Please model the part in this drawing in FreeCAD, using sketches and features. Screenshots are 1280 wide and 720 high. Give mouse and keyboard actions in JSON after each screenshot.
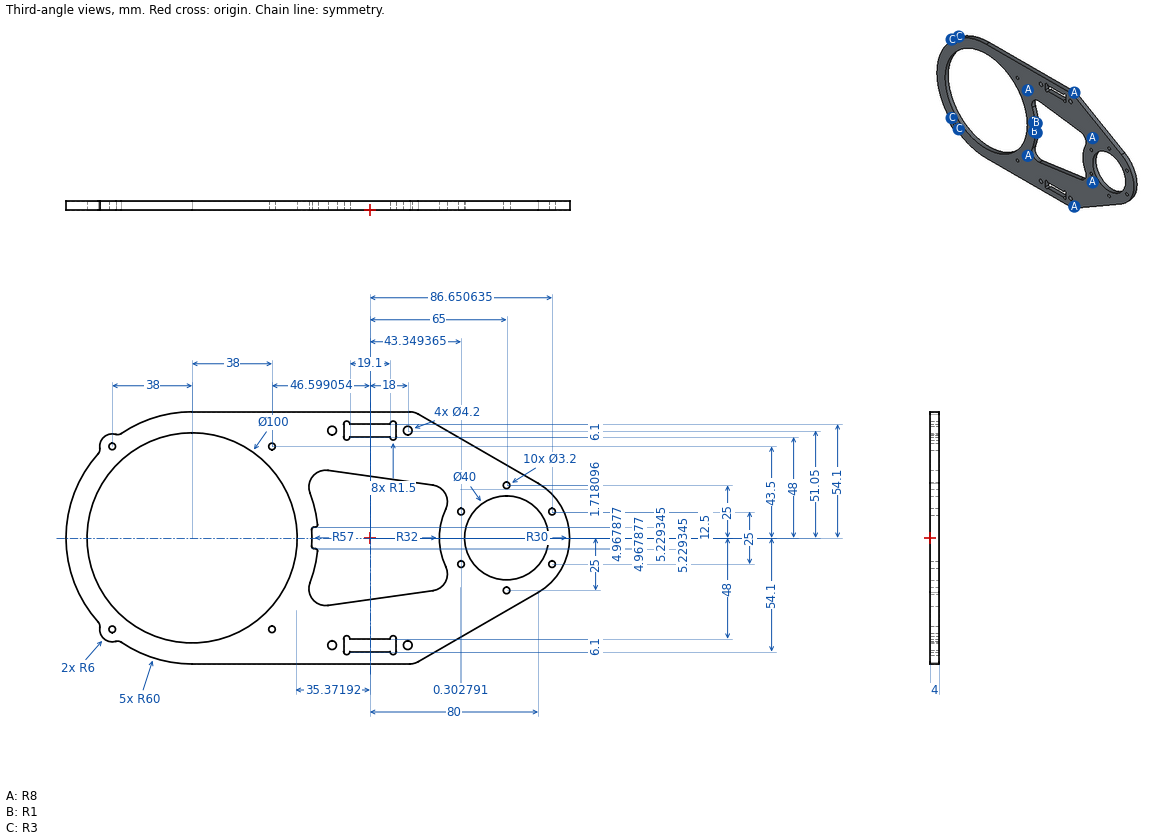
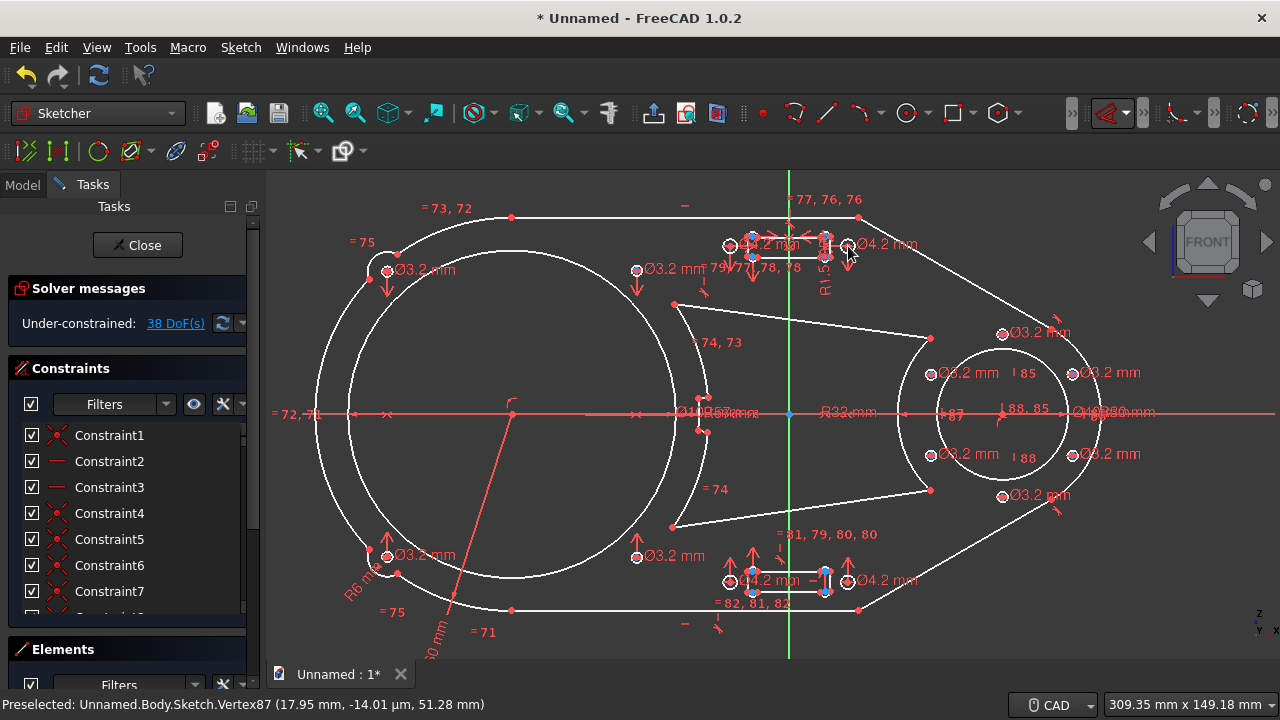
{"action": "left_click", "coordinate": [1128, 114]}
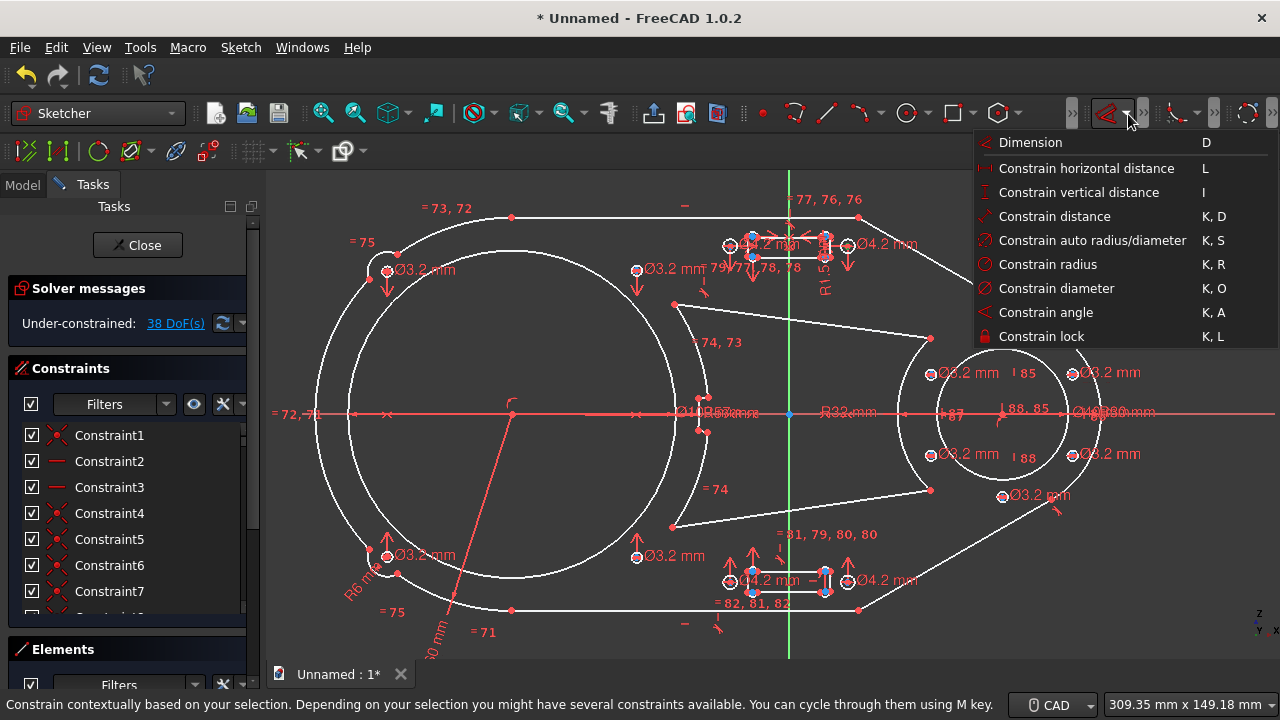
{"action": "left_click", "coordinate": [1126, 168]}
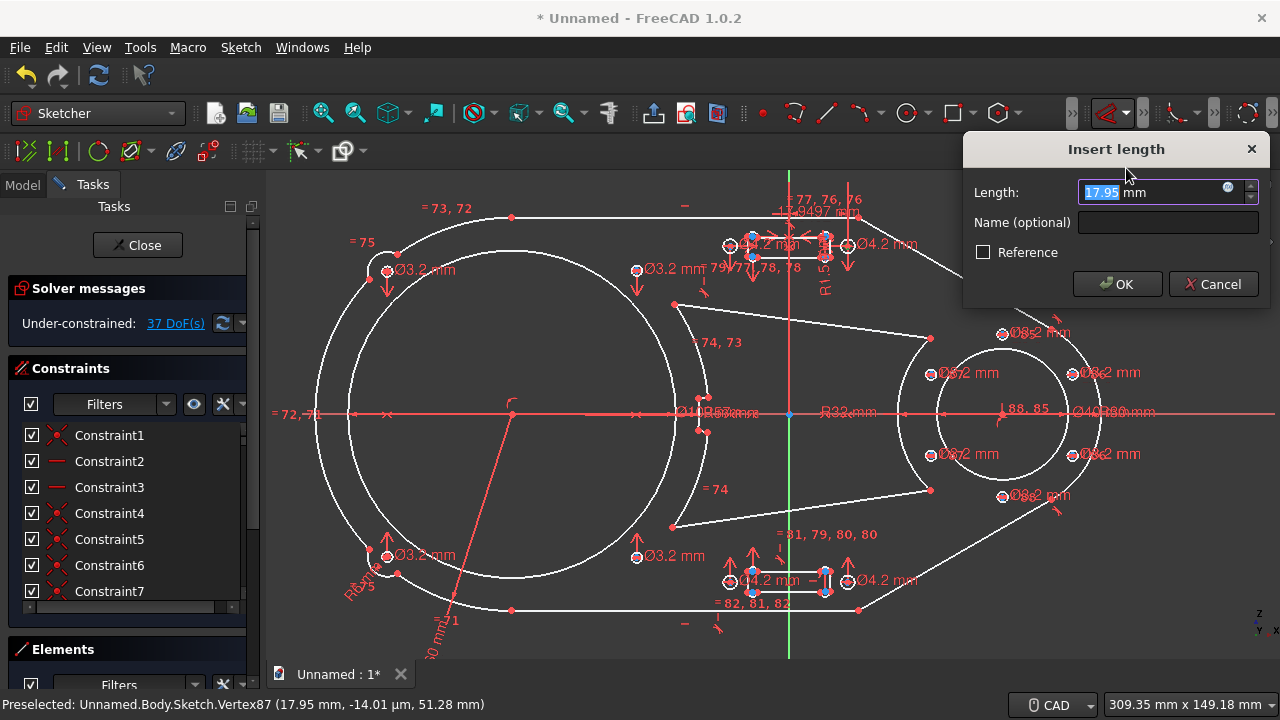
{"action": "type", "text": "18"}
{"action": "key", "text": "Return"}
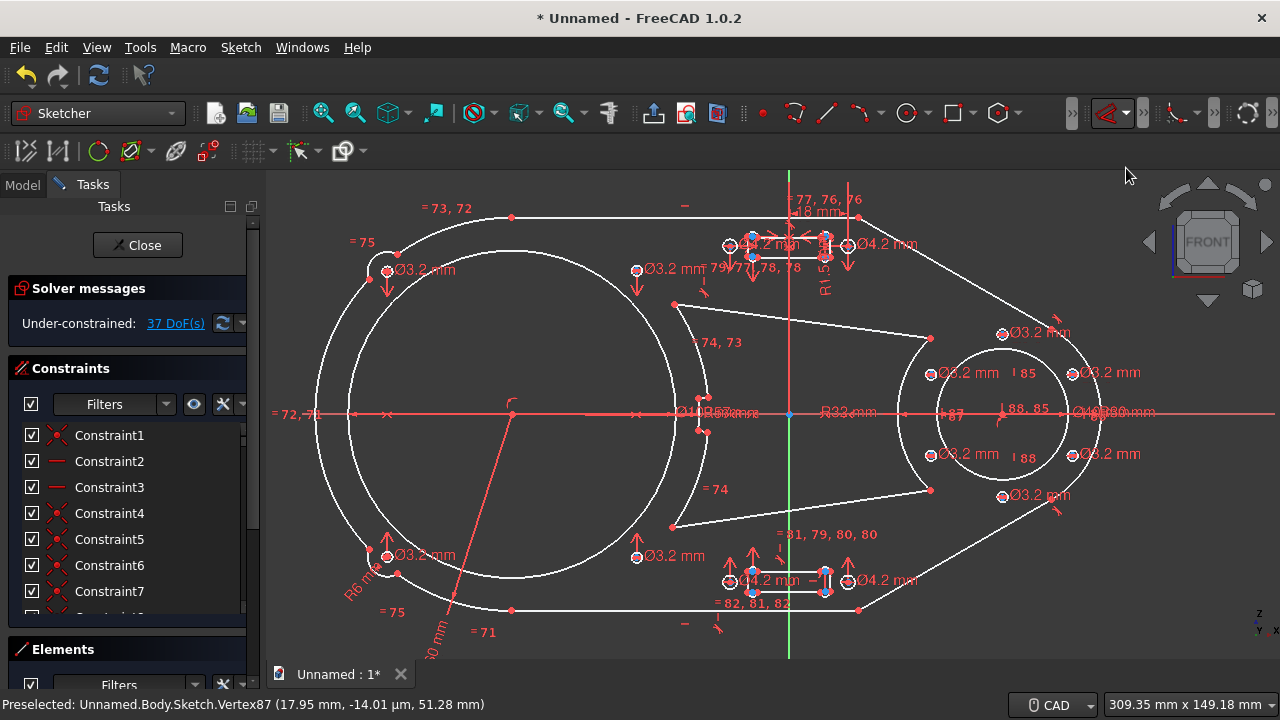
{"action": "left_click", "coordinate": [1003, 335]}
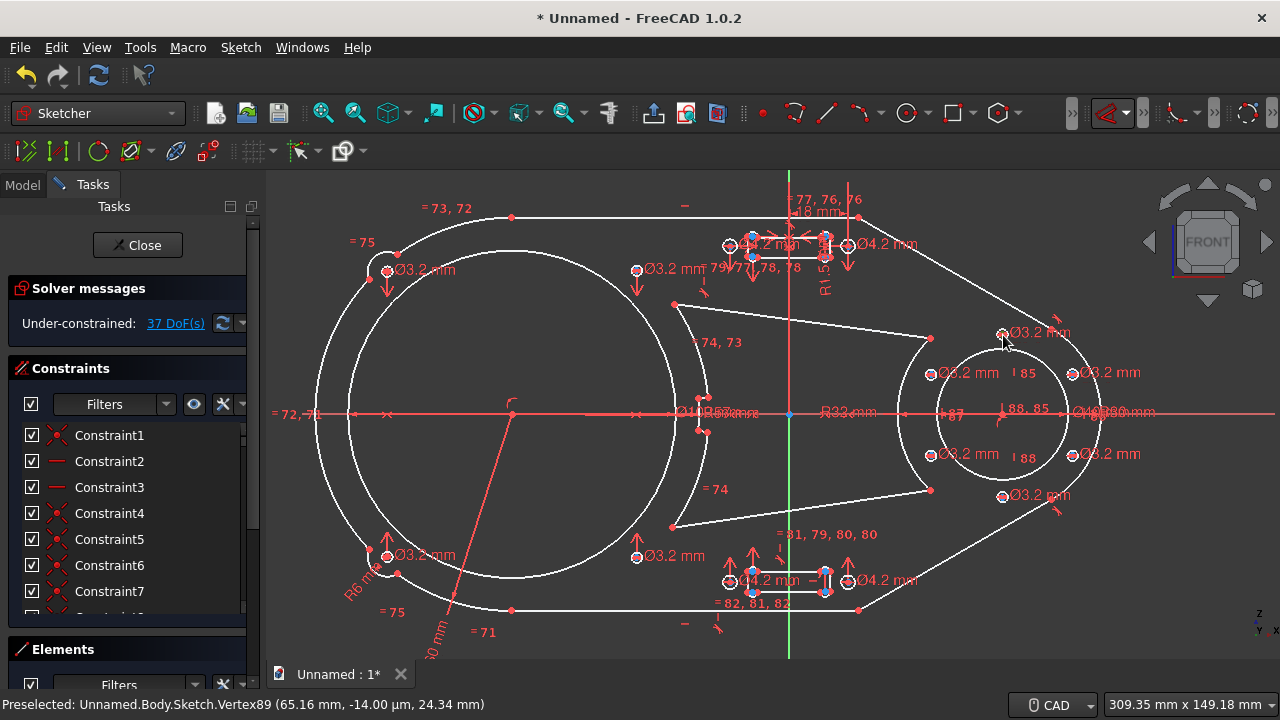
{"action": "left_click", "coordinate": [1128, 114]}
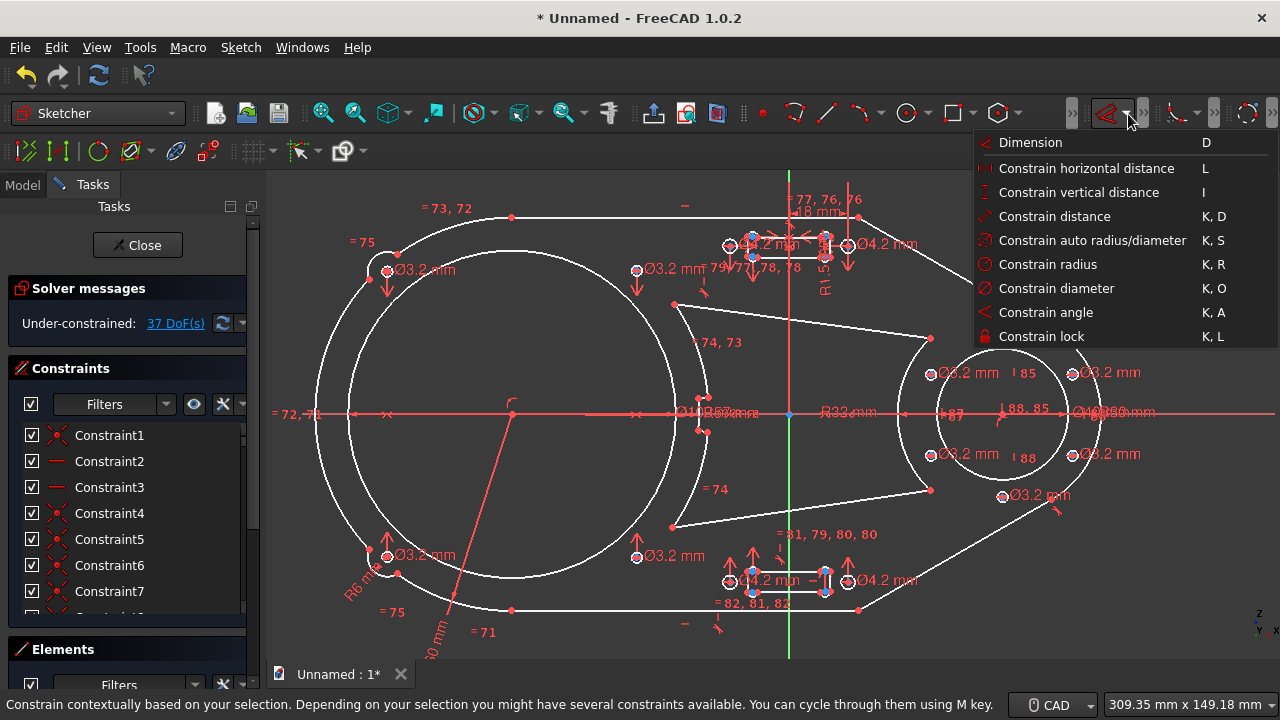
{"action": "left_click", "coordinate": [1126, 168]}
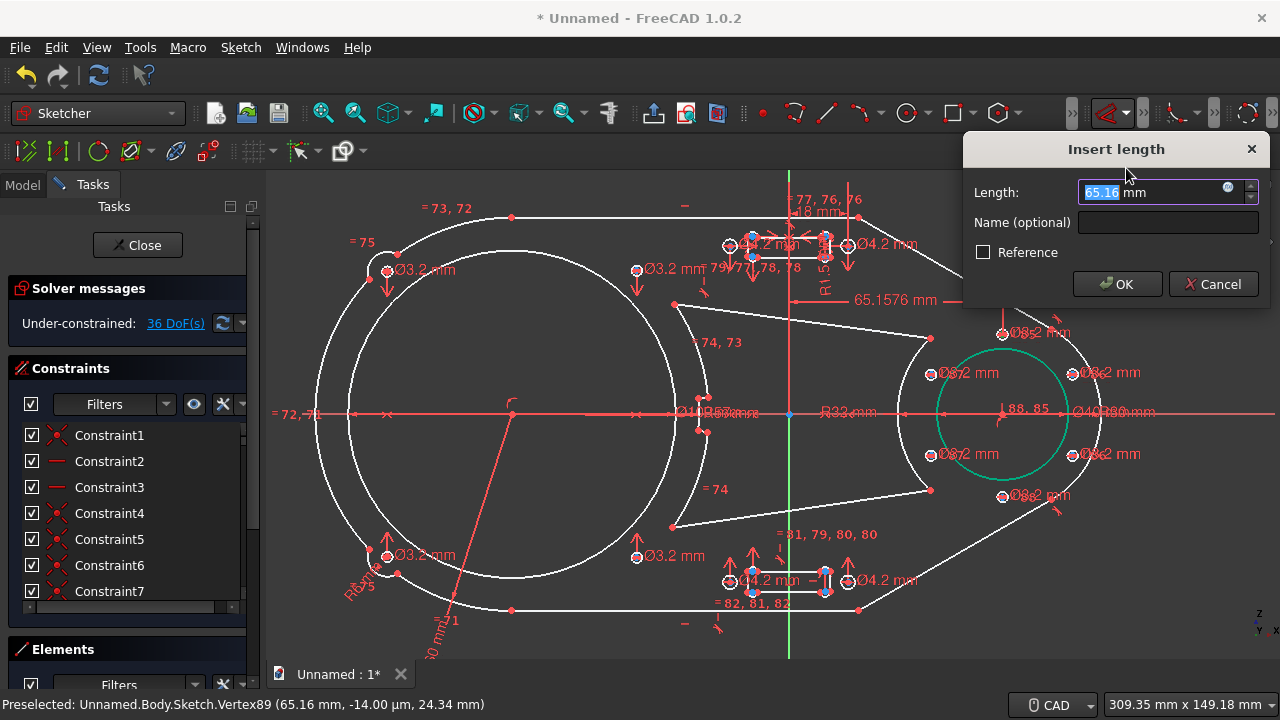
{"action": "type", "text": "65"}
{"action": "key", "text": "Return"}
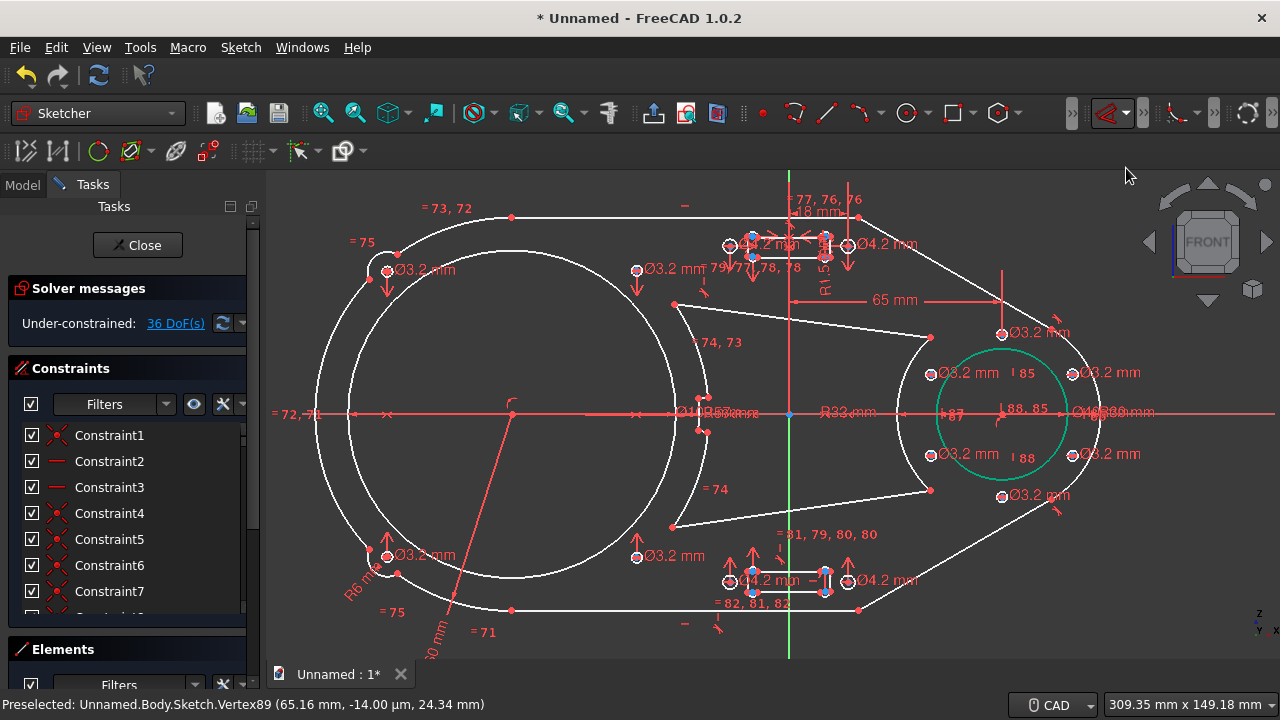
{"action": "left_click", "coordinate": [1002, 335]}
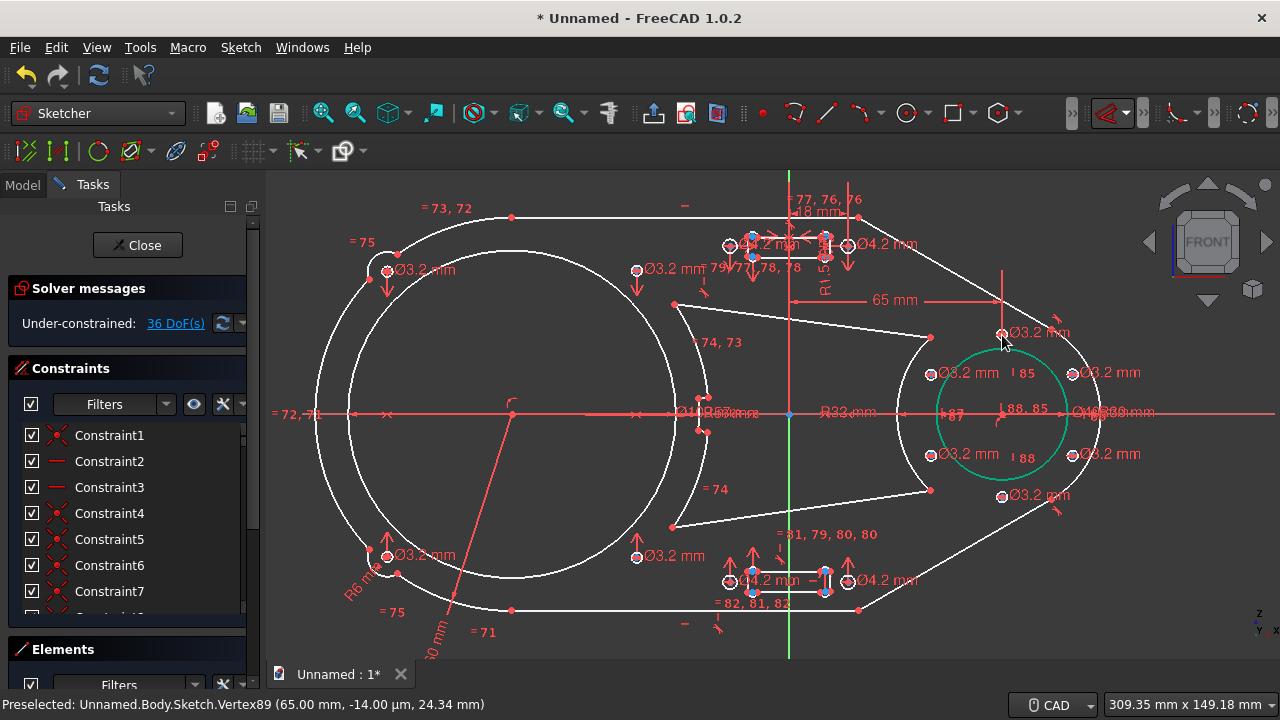
{"action": "key", "text": "i"}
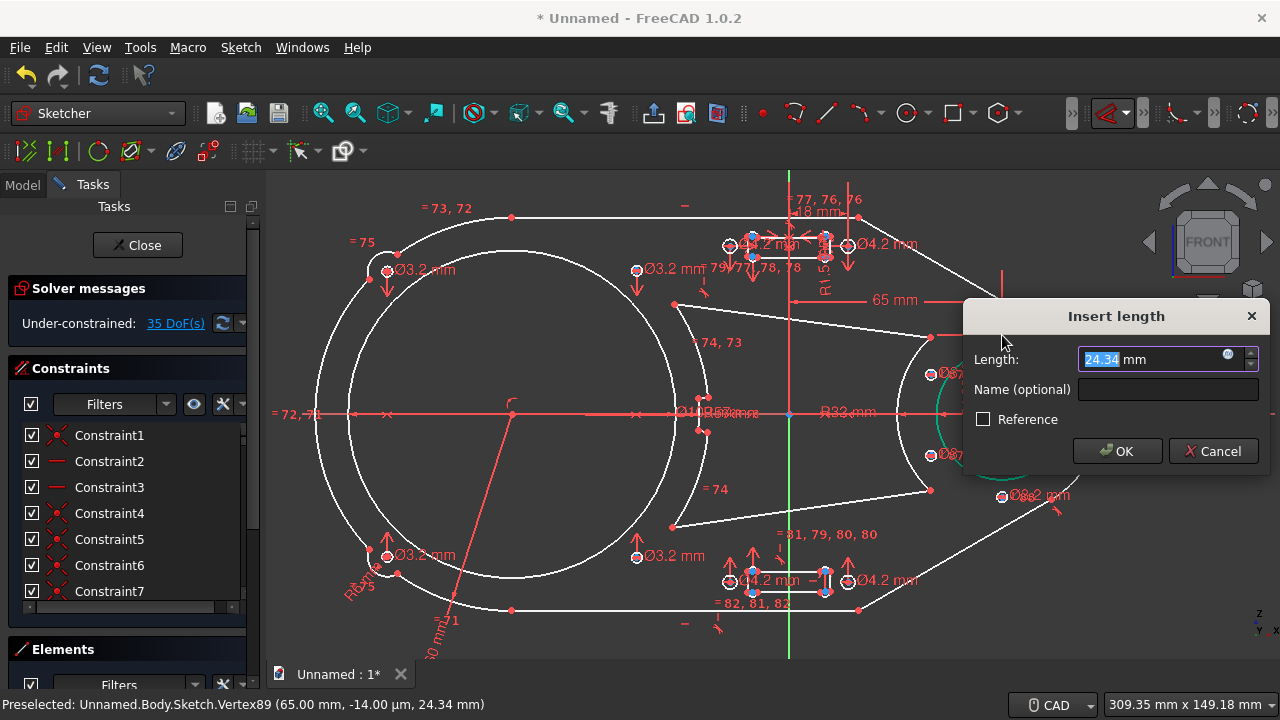
{"action": "type", "text": "25"}
{"action": "key", "text": "Return"}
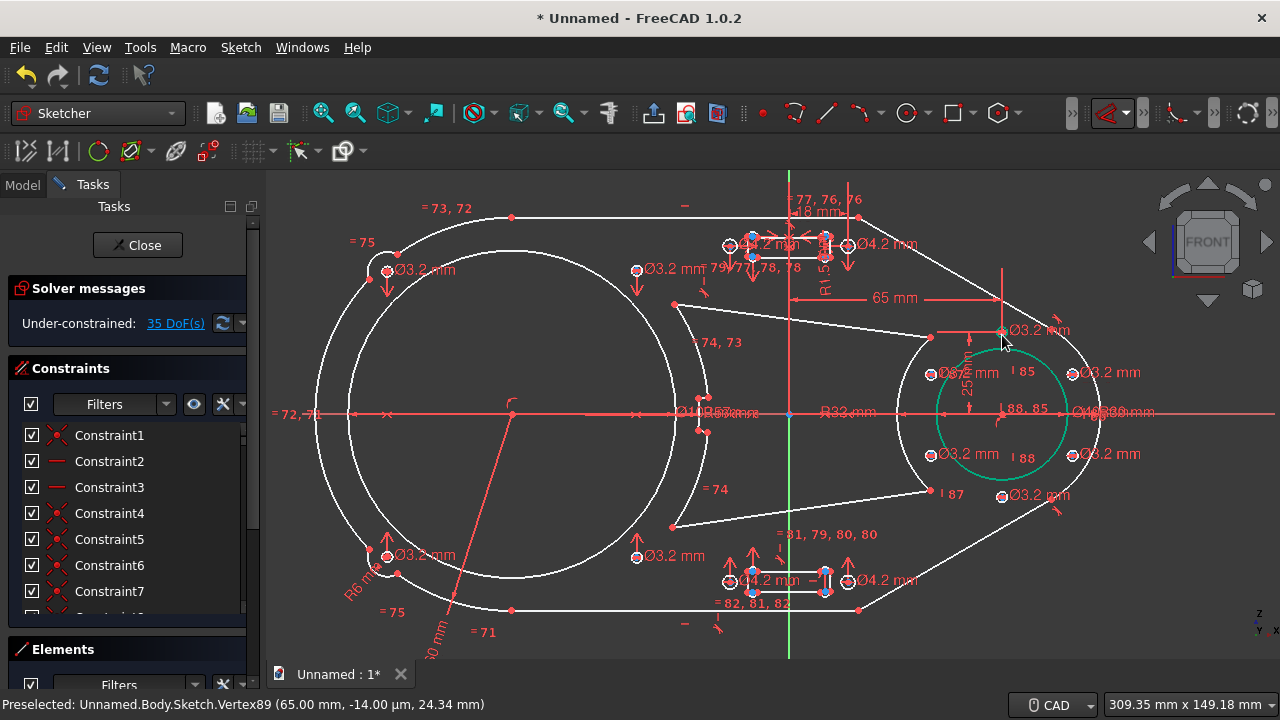
{"action": "left_click", "coordinate": [1002, 497]}